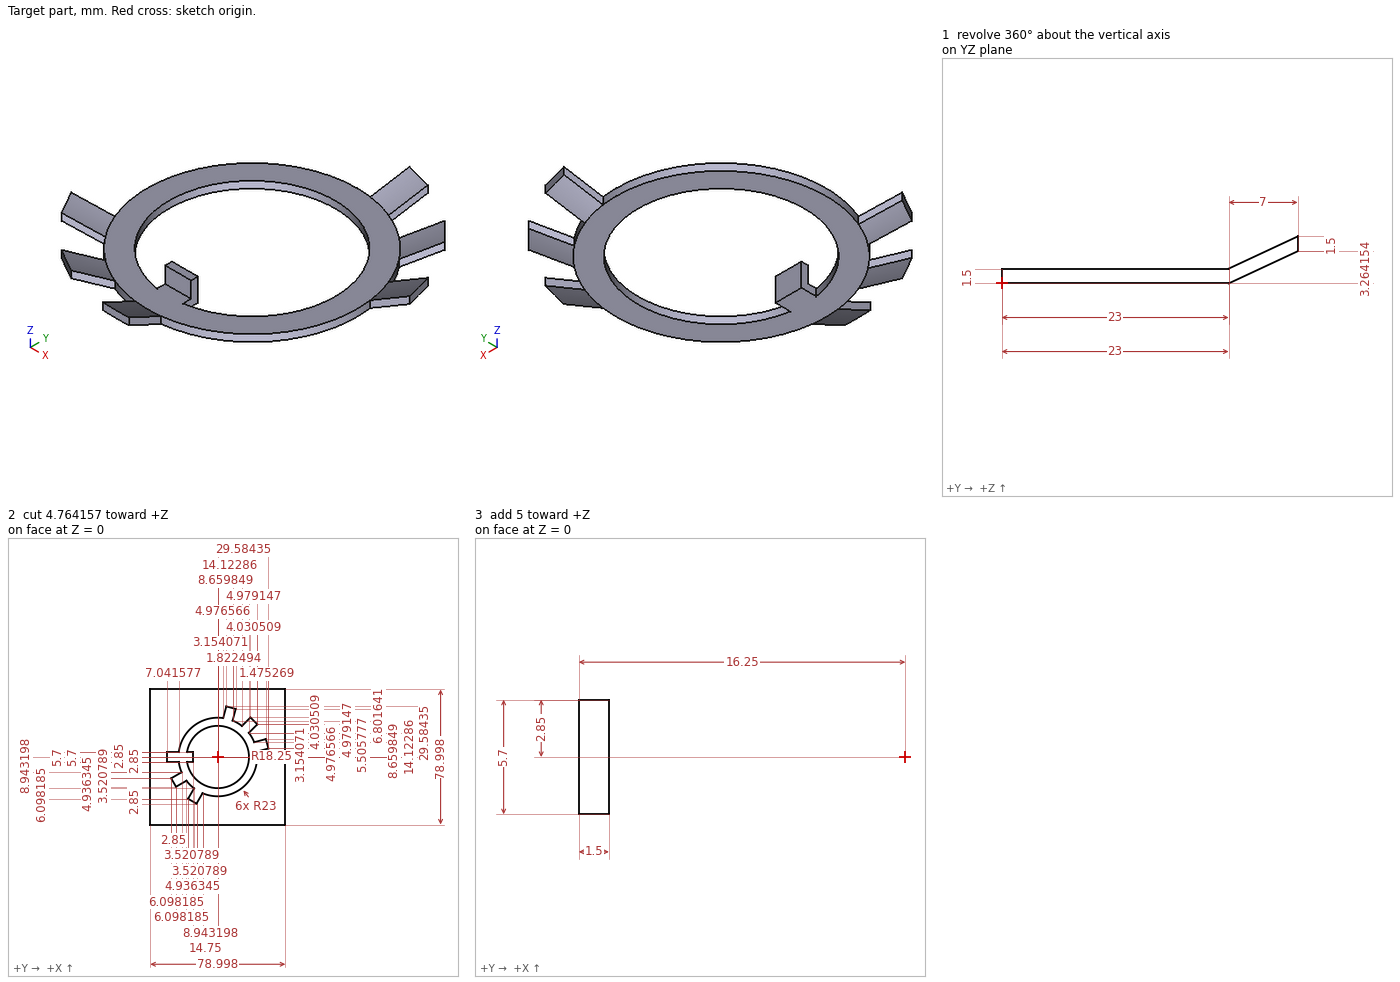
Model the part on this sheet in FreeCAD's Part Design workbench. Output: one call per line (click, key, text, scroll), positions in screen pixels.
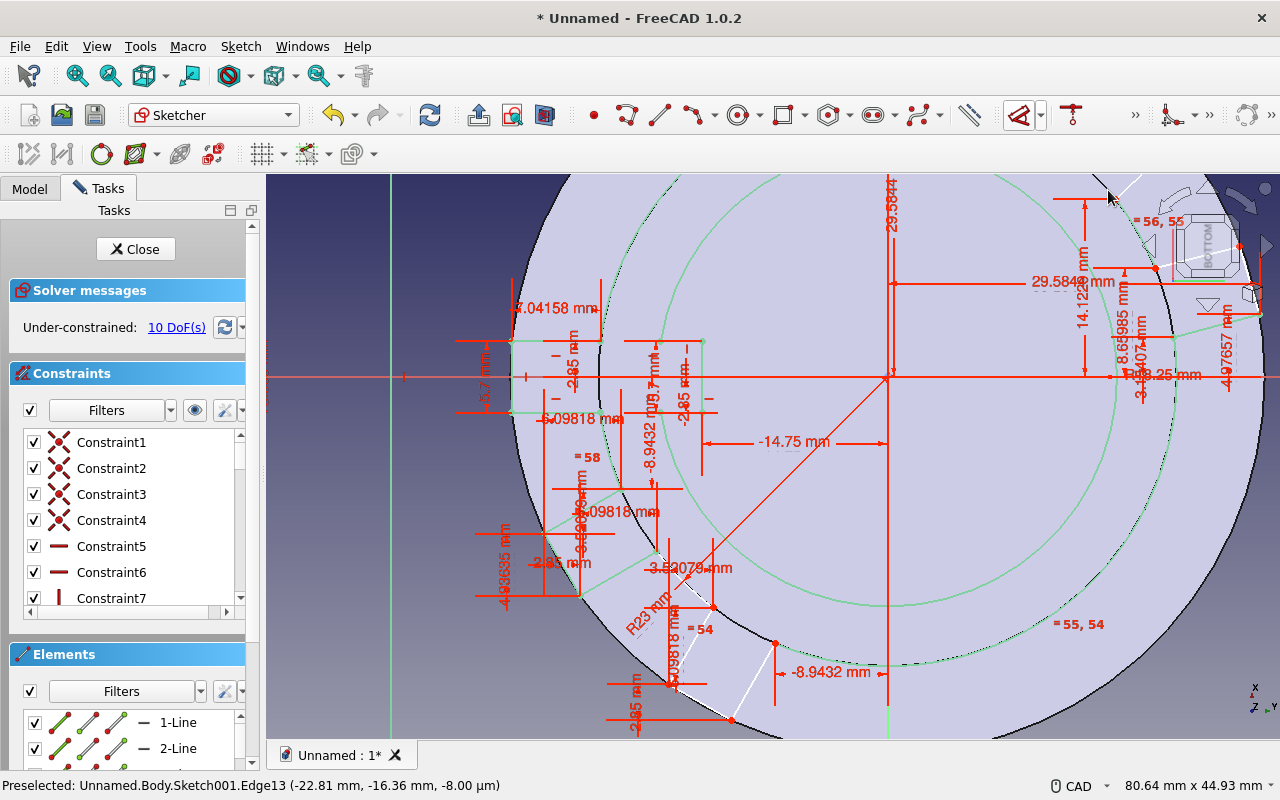
click(688, 695)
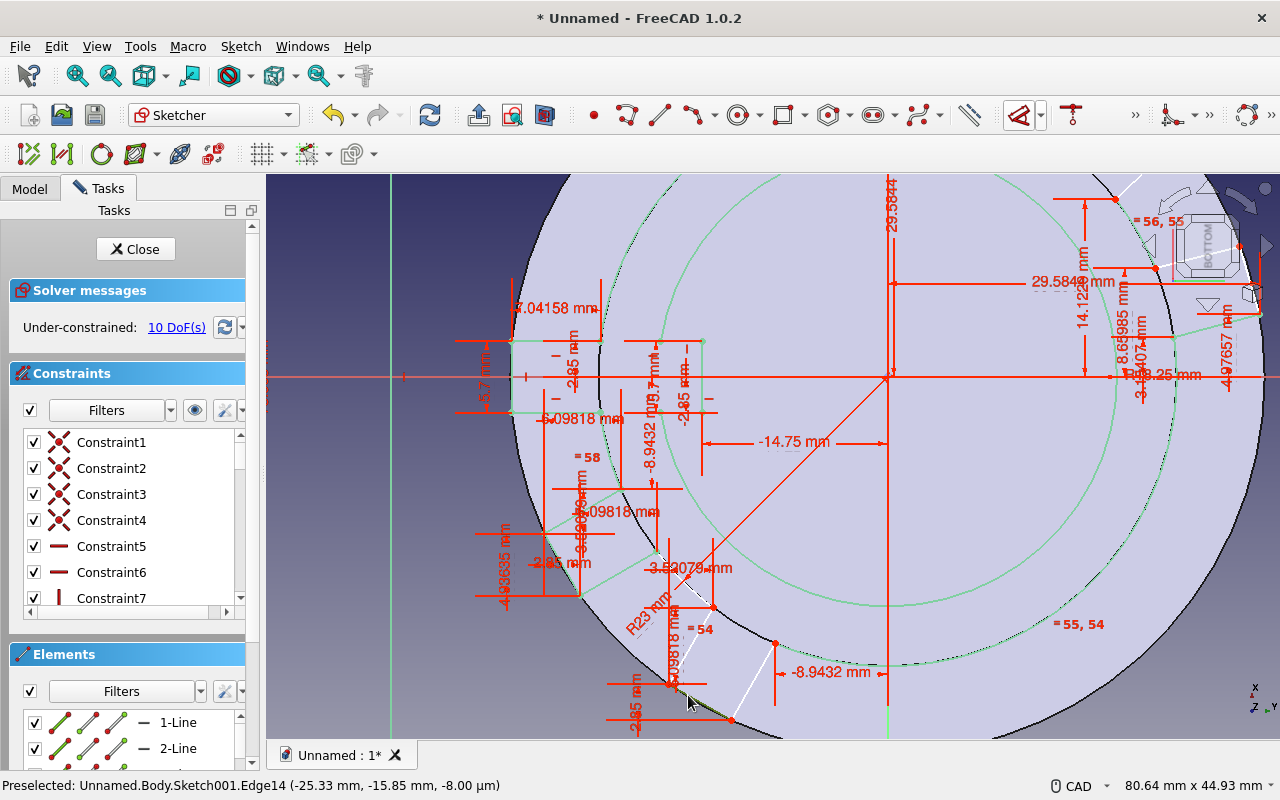
click(1040, 116)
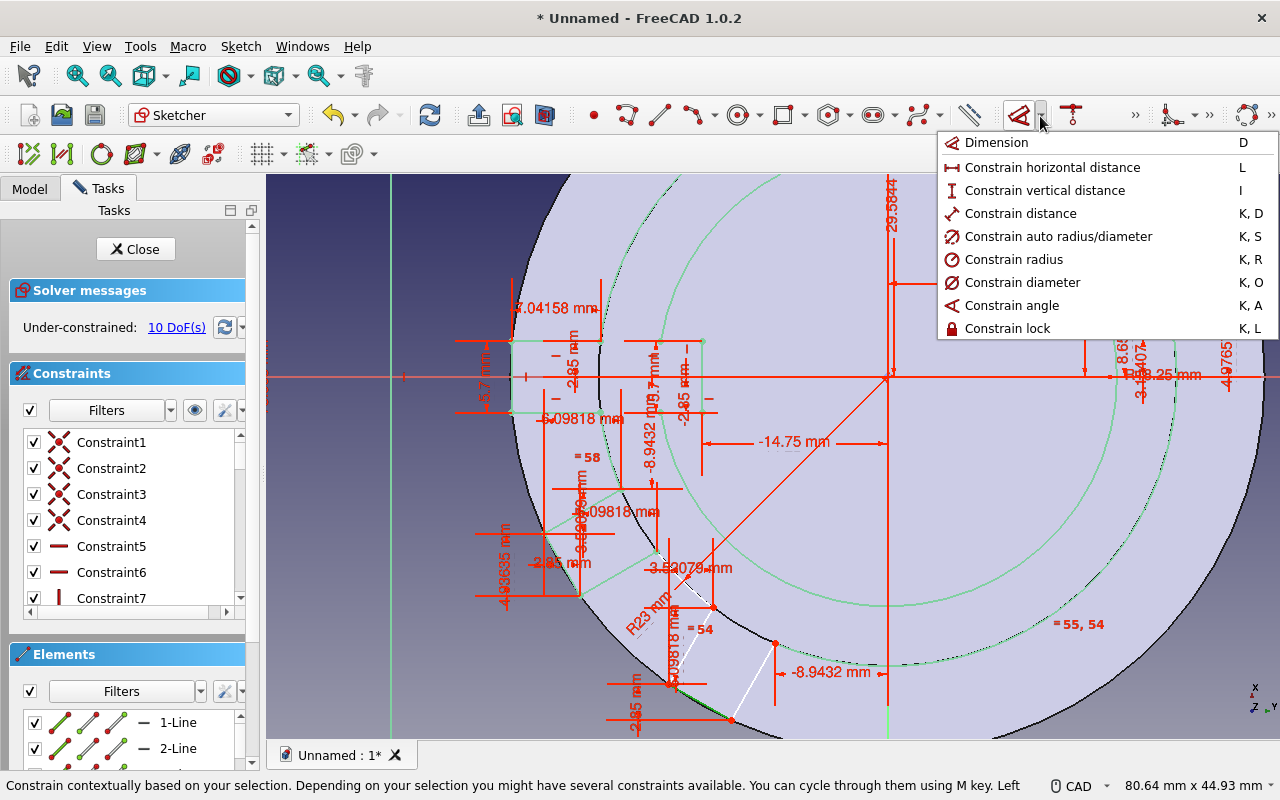
click(1108, 168)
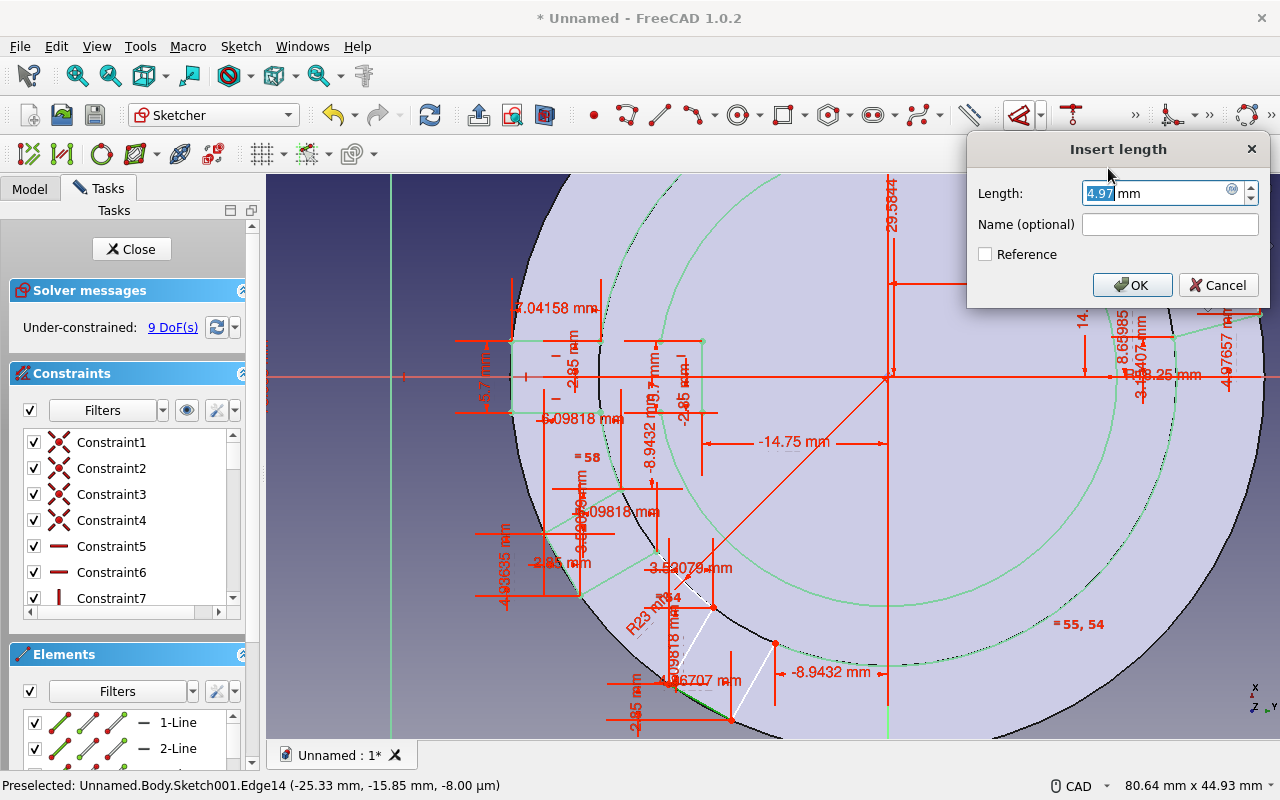
text(4.936345)
key(Return)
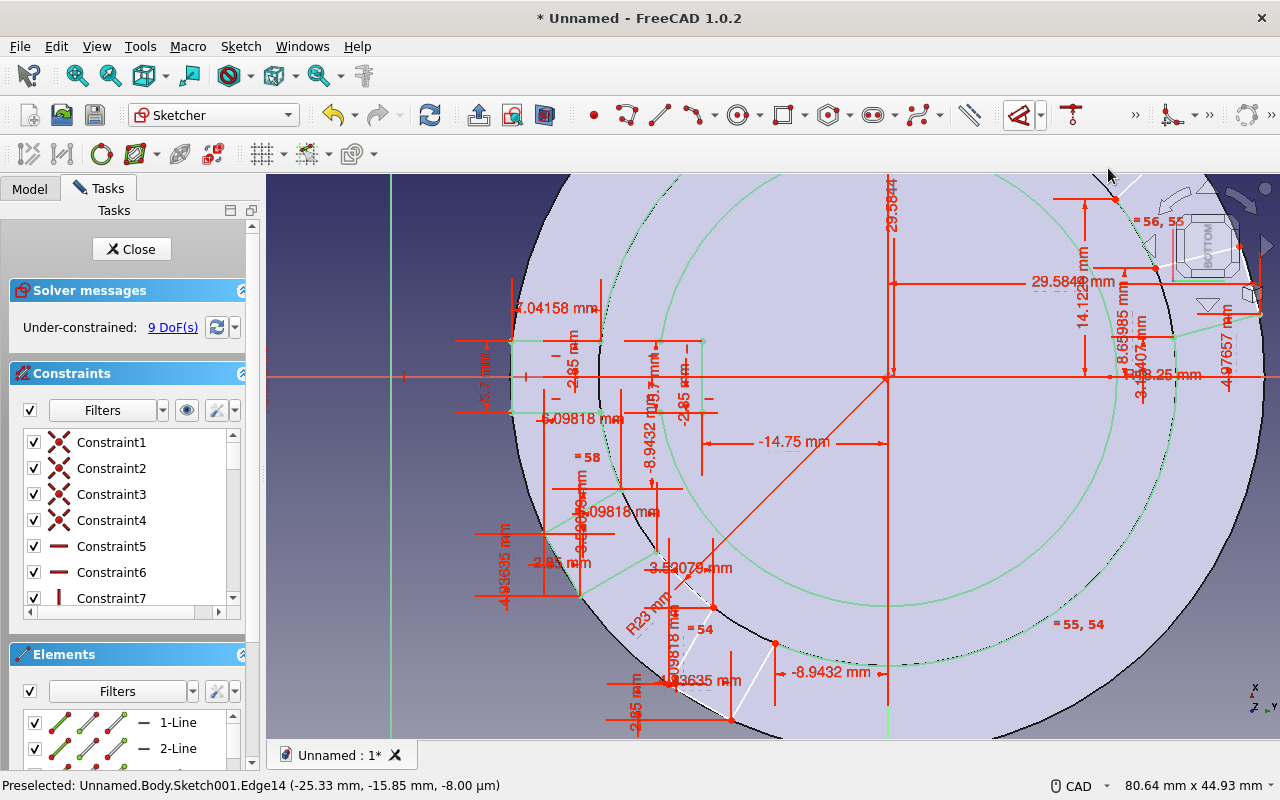
click(744, 697)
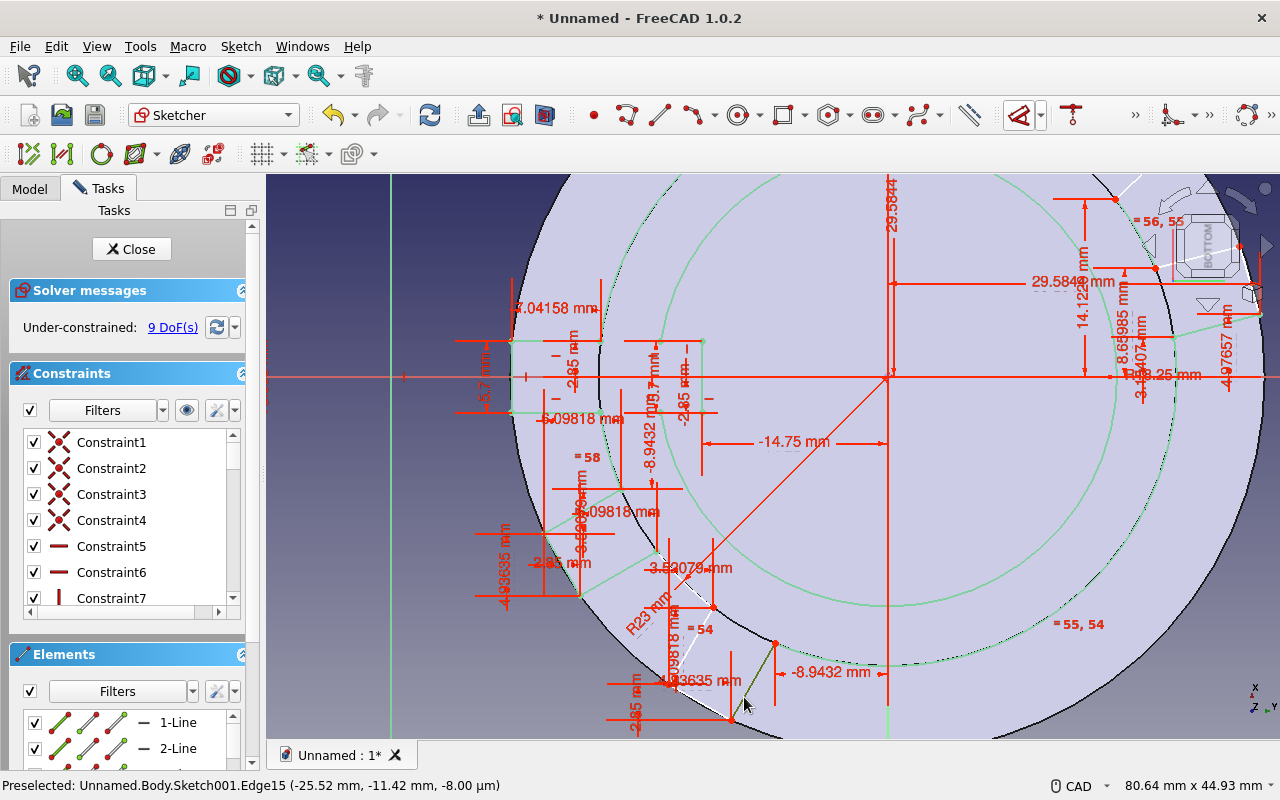
click(1040, 116)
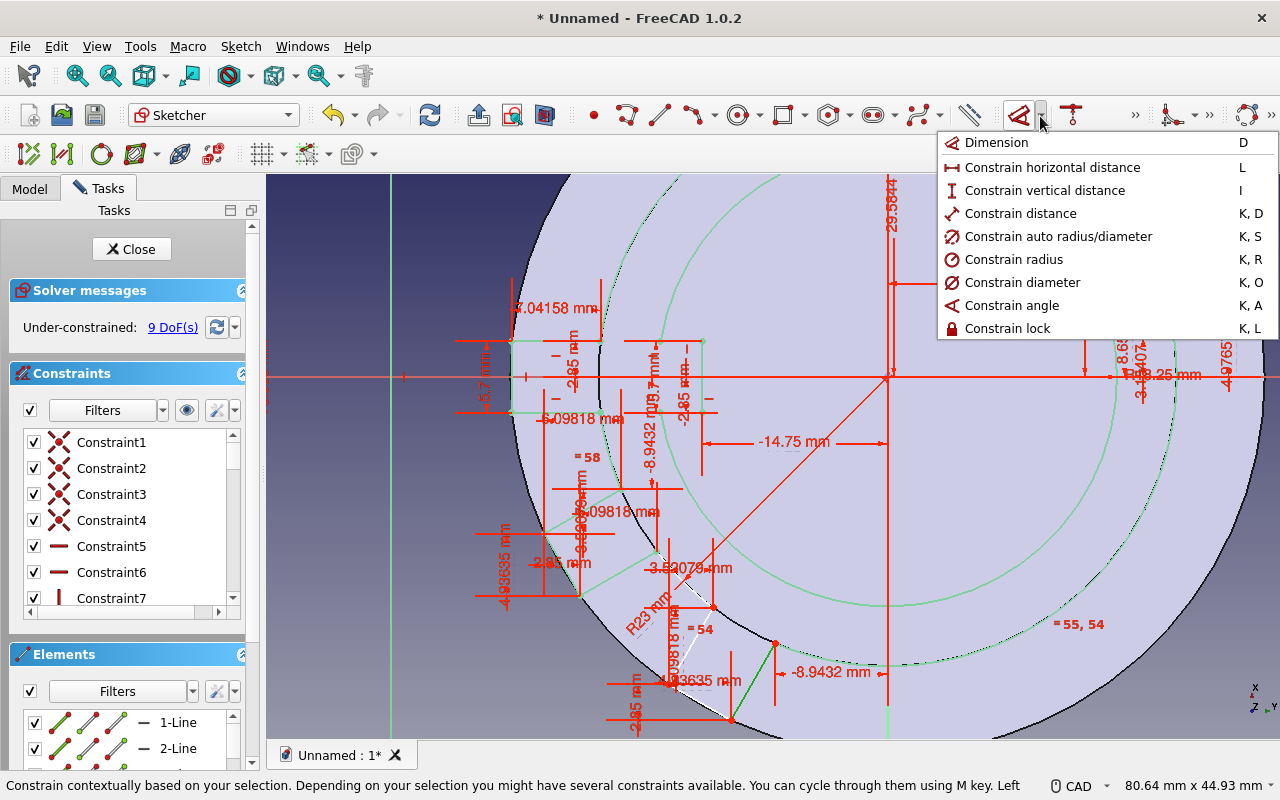
click(1108, 168)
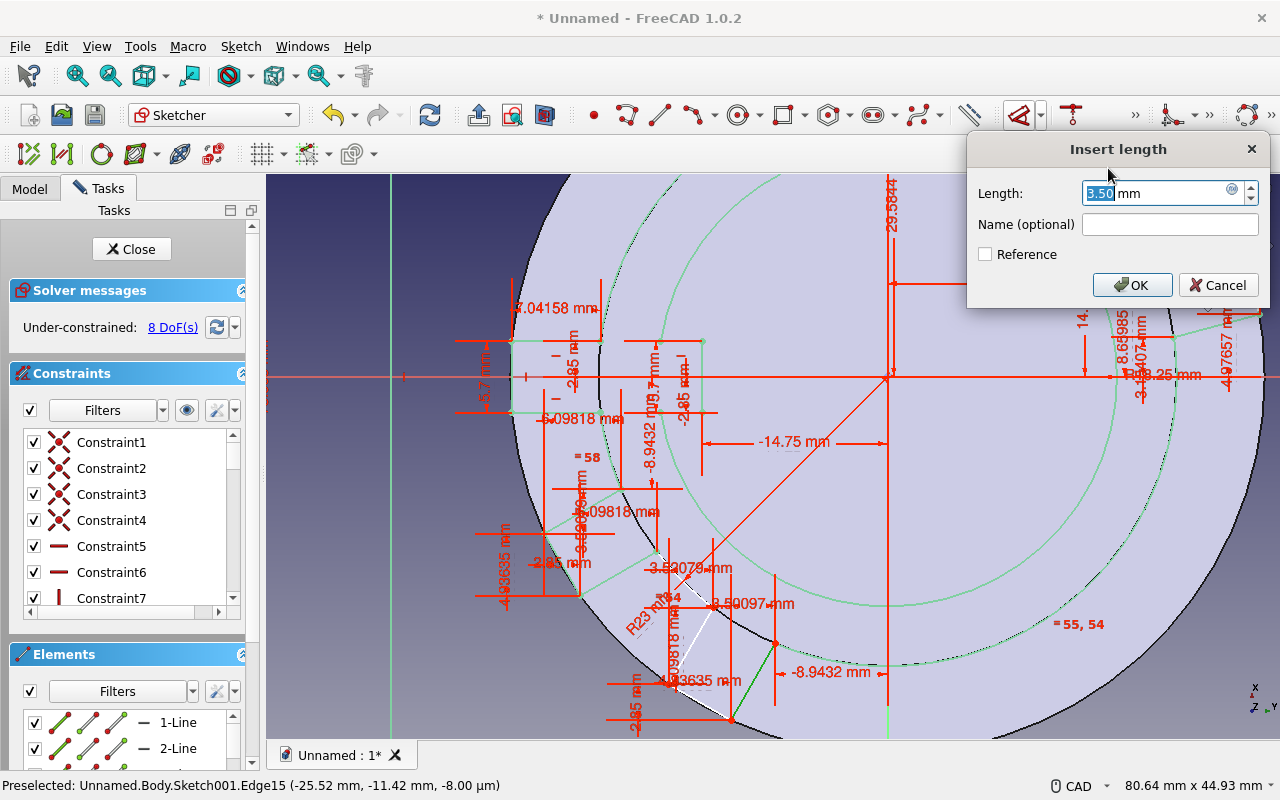
text(3.520789)
key(Return)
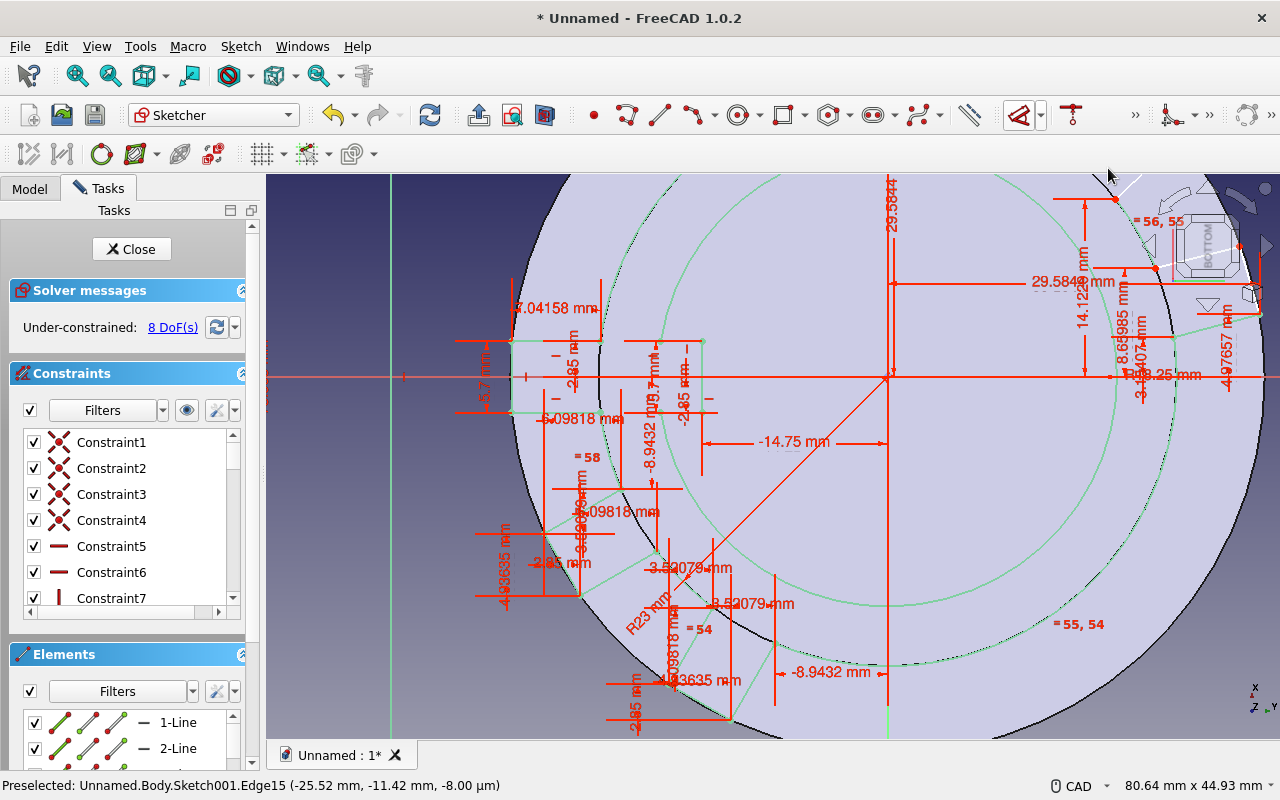
scroll(598, 503, down, 5)